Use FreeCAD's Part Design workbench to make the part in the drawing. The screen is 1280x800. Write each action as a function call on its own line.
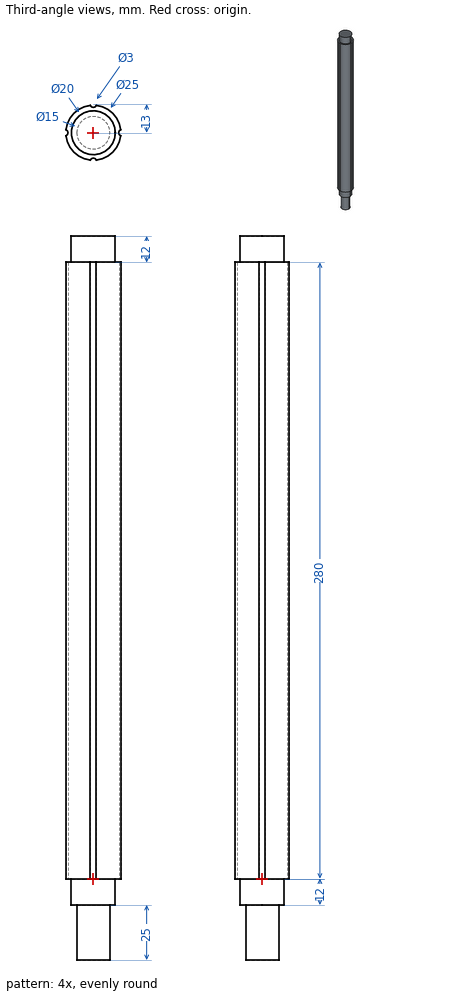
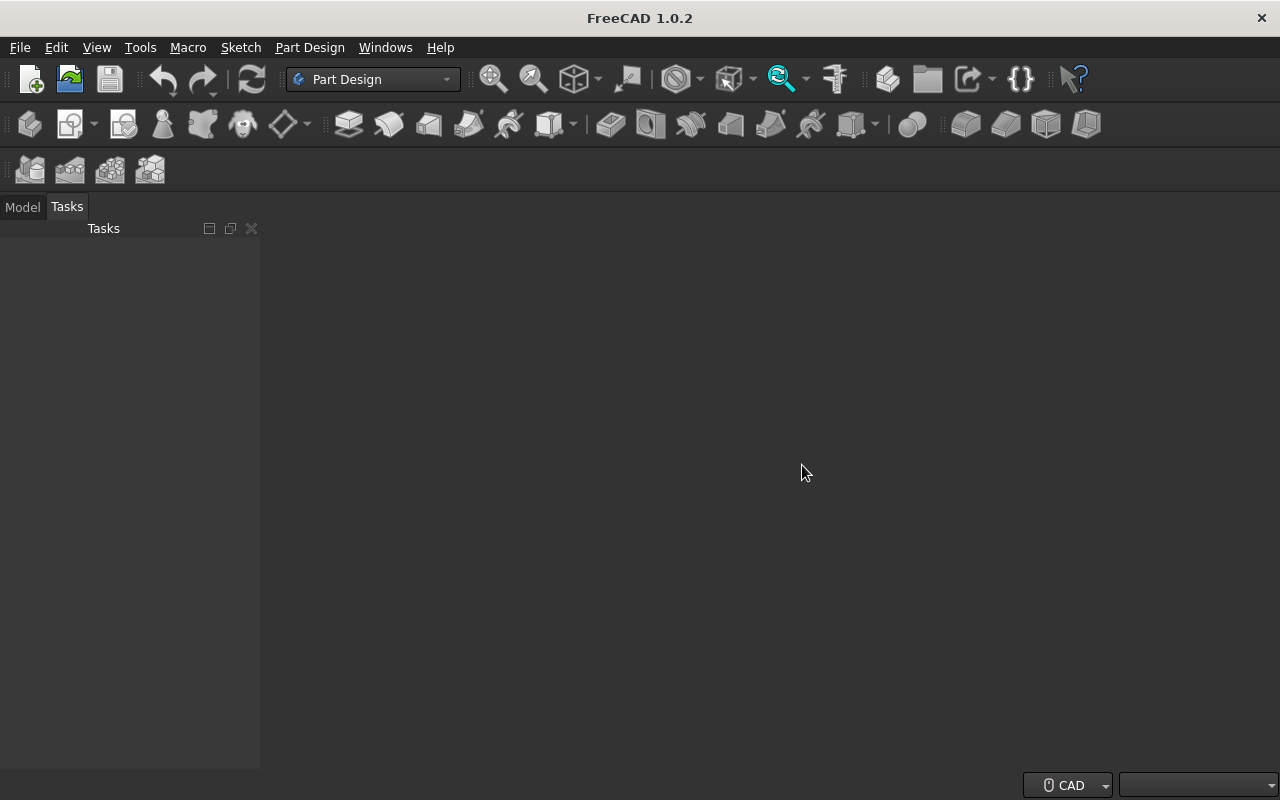
key(ctrl+n)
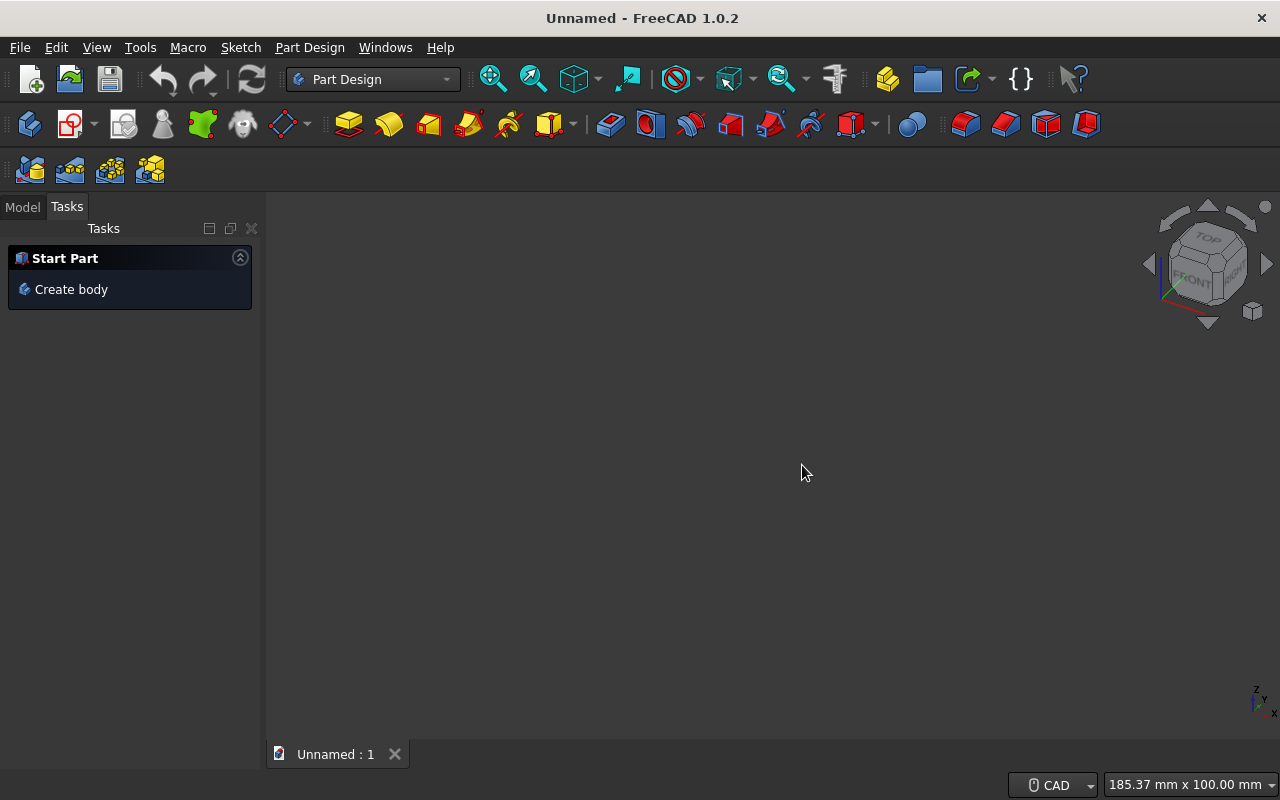
click(70, 124)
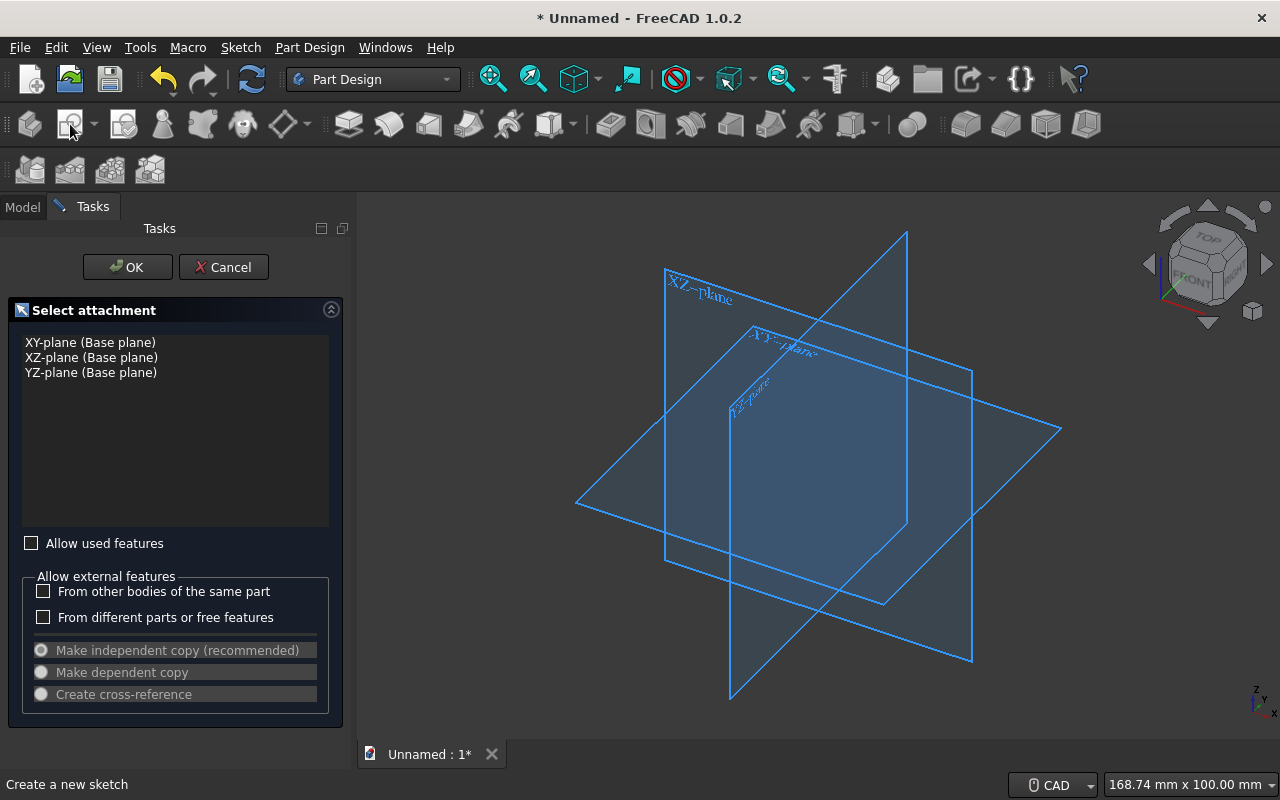
click(82, 342)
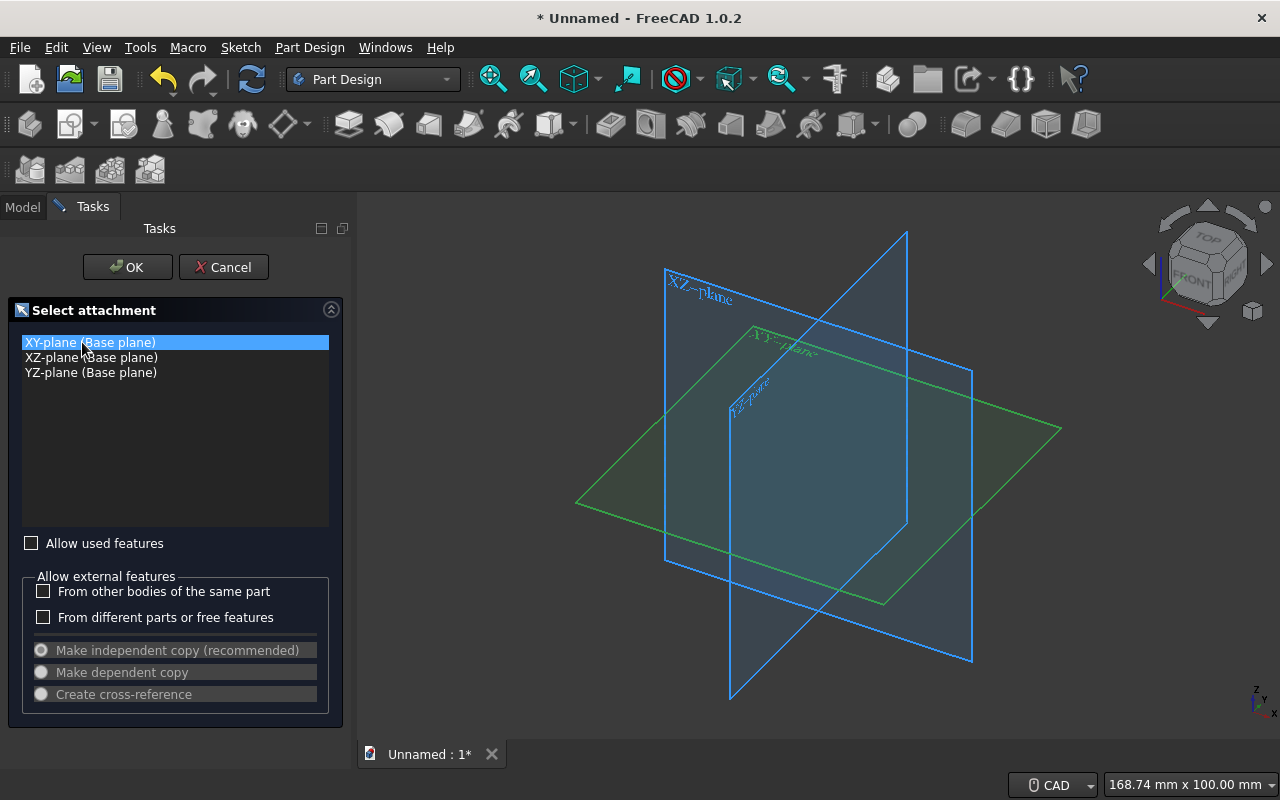
click(128, 267)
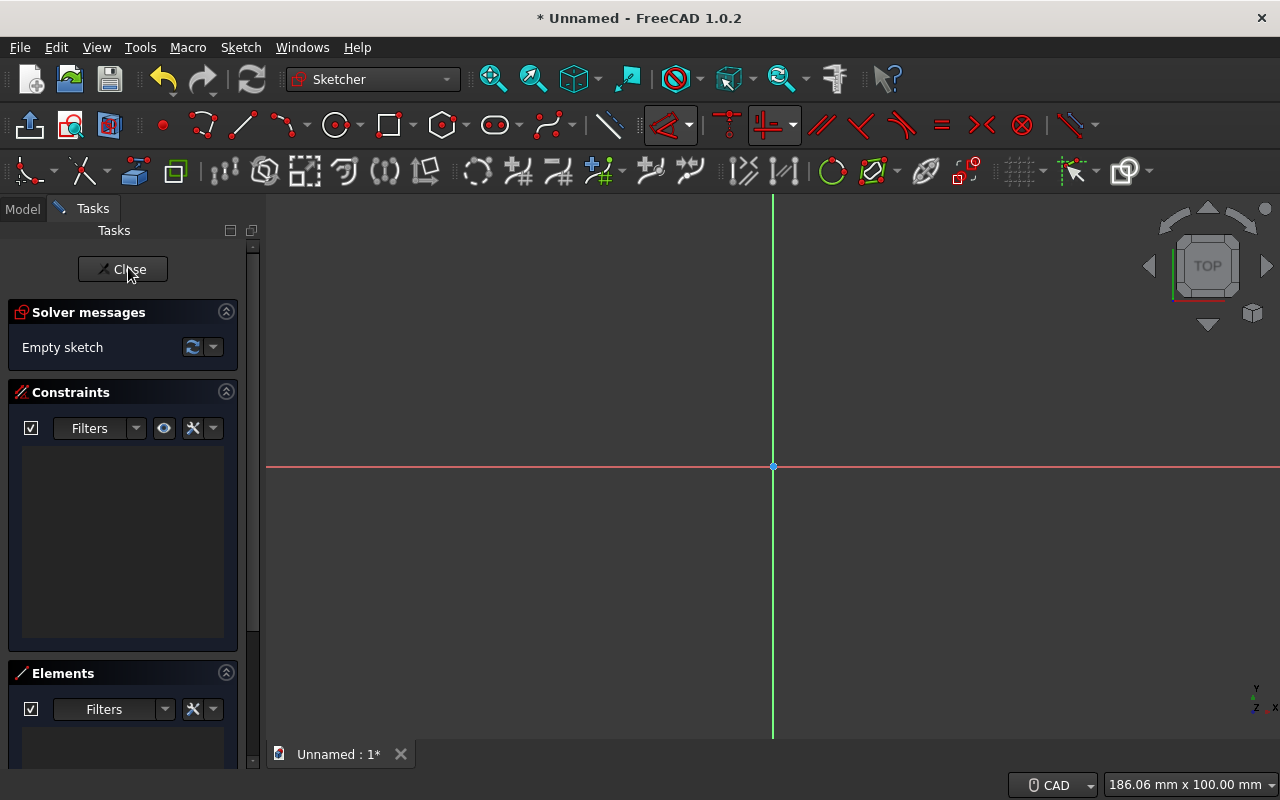
scroll(813, 466, up, 5)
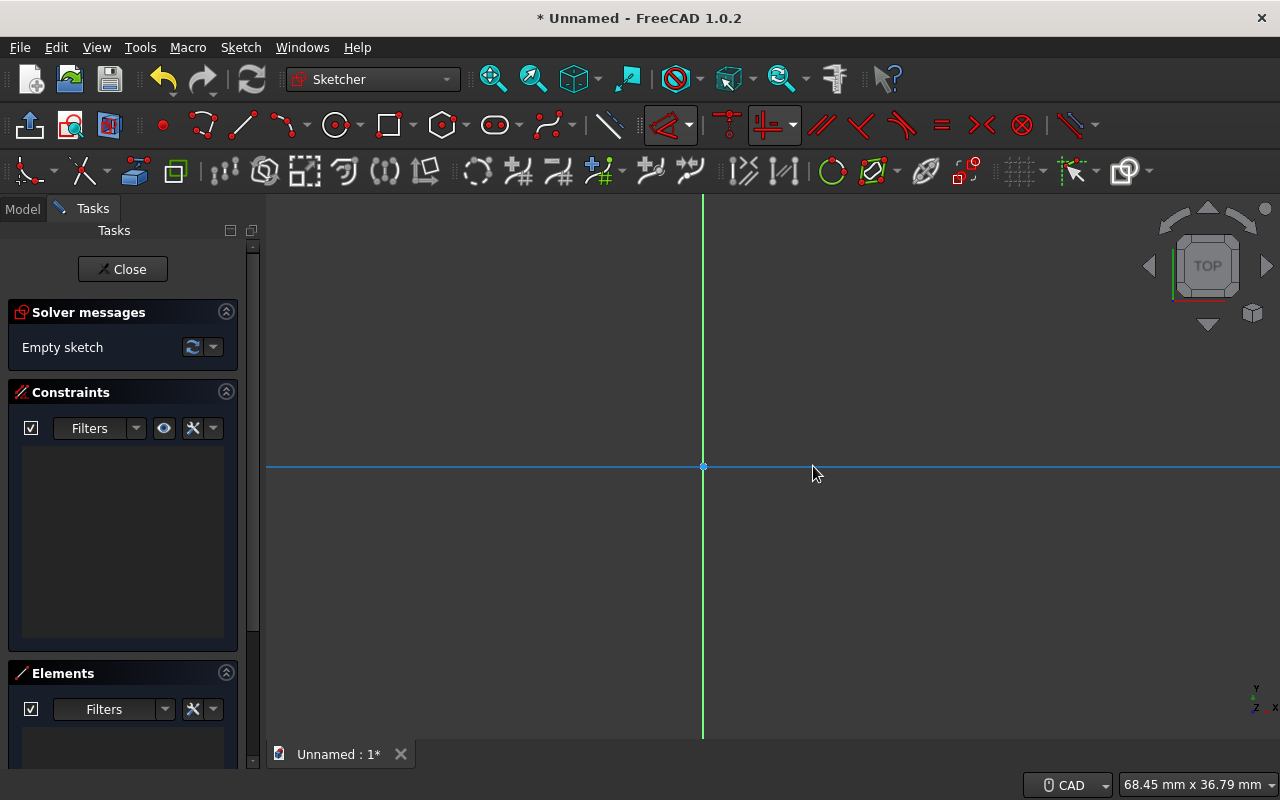
key(g)
key(c)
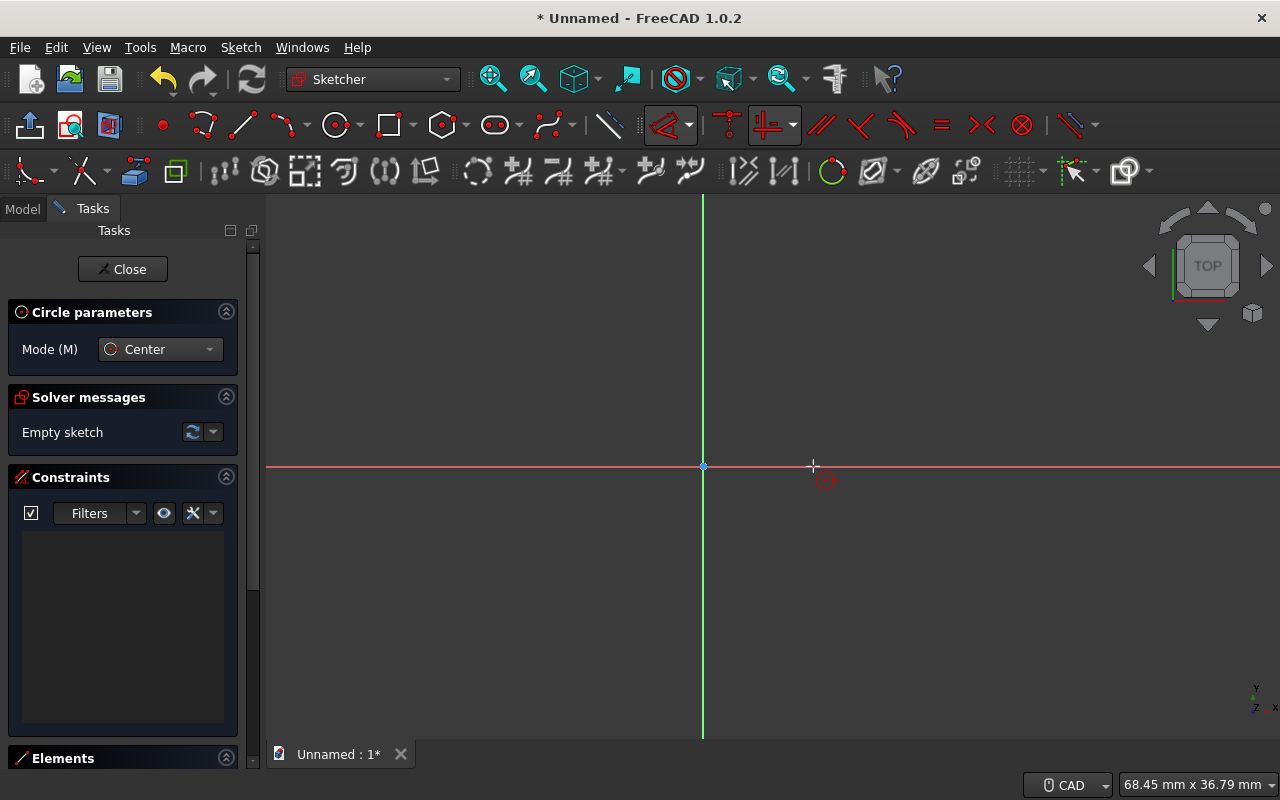
click(703, 466)
click(834, 336)
key(Escape)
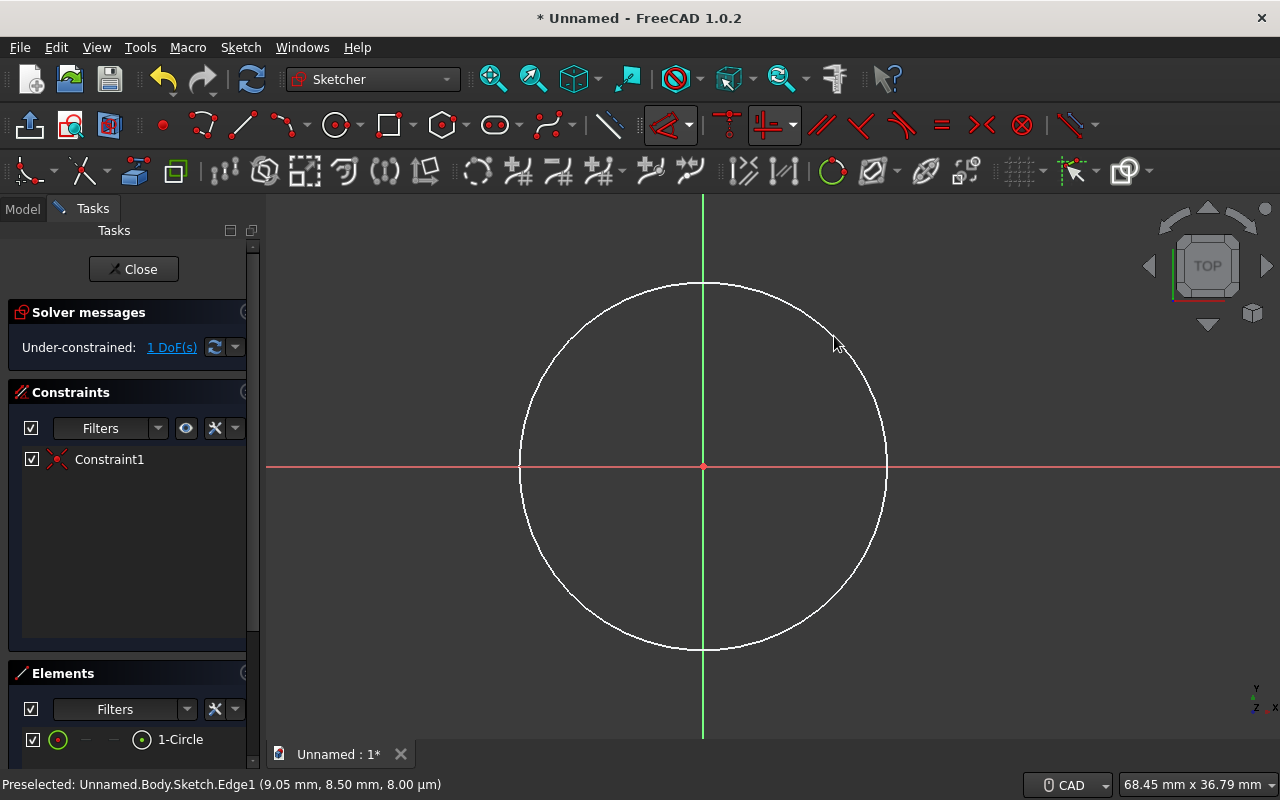
key(d)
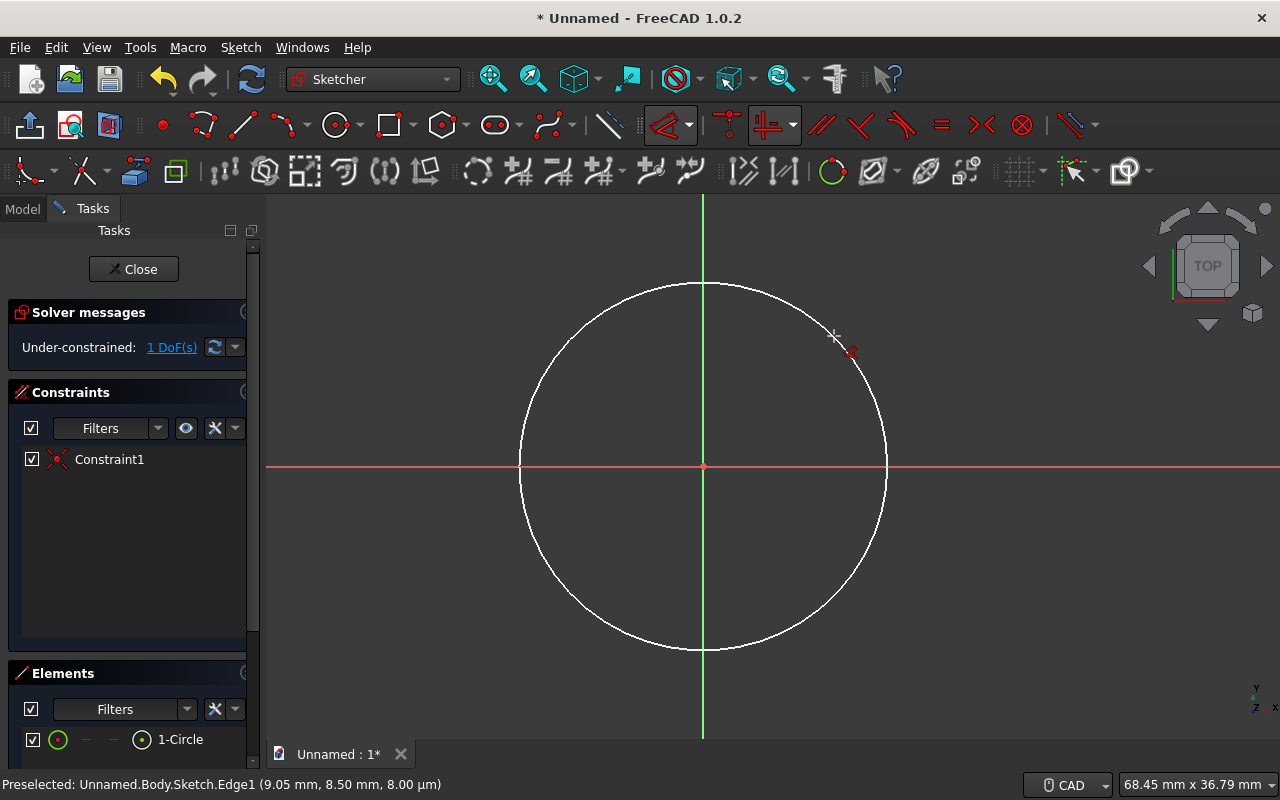
click(833, 336)
click(856, 313)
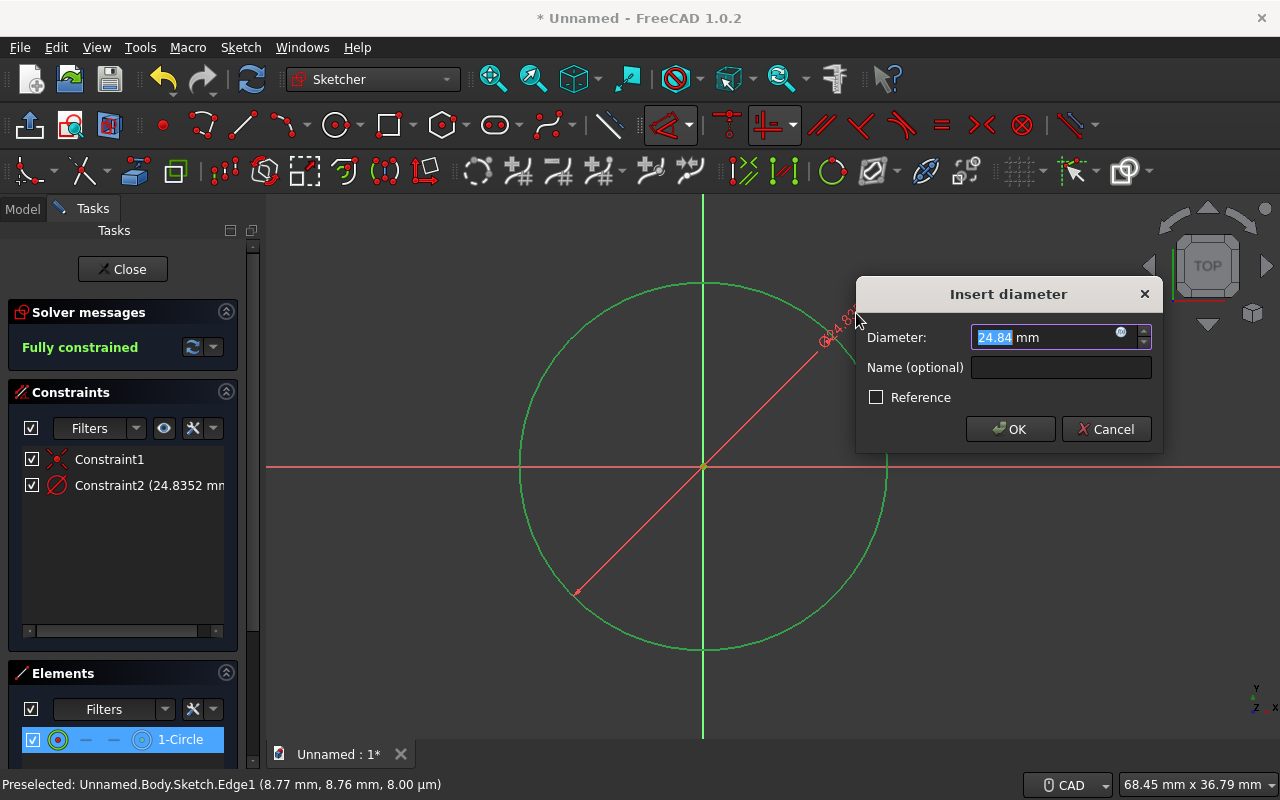
text(25)
key(Return)
key(Escape)